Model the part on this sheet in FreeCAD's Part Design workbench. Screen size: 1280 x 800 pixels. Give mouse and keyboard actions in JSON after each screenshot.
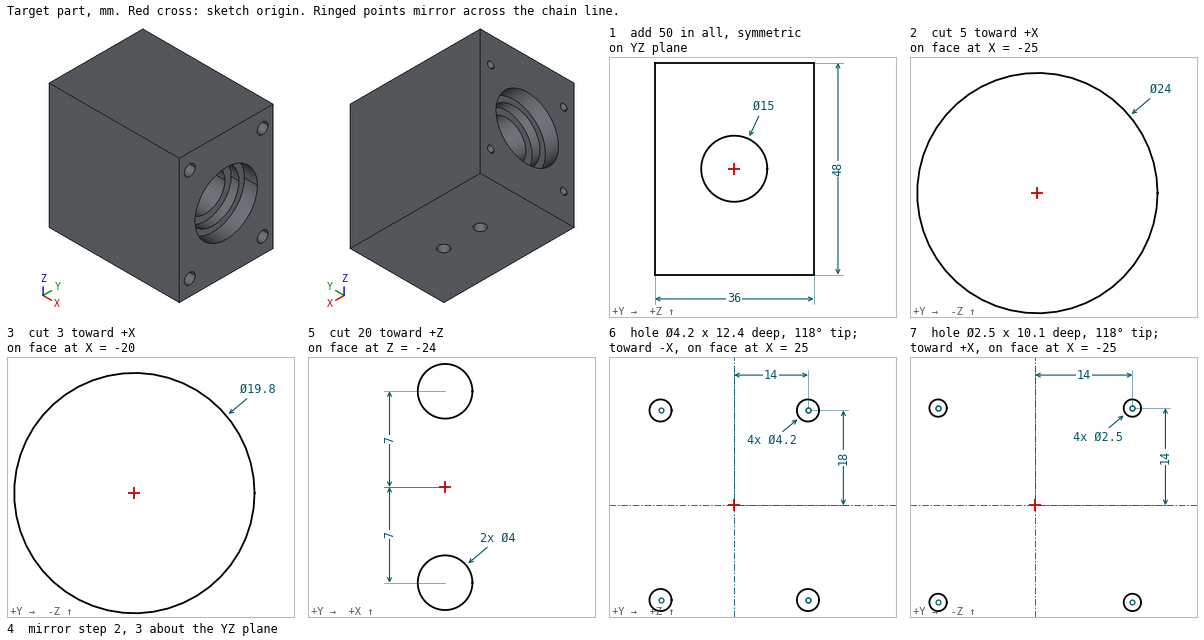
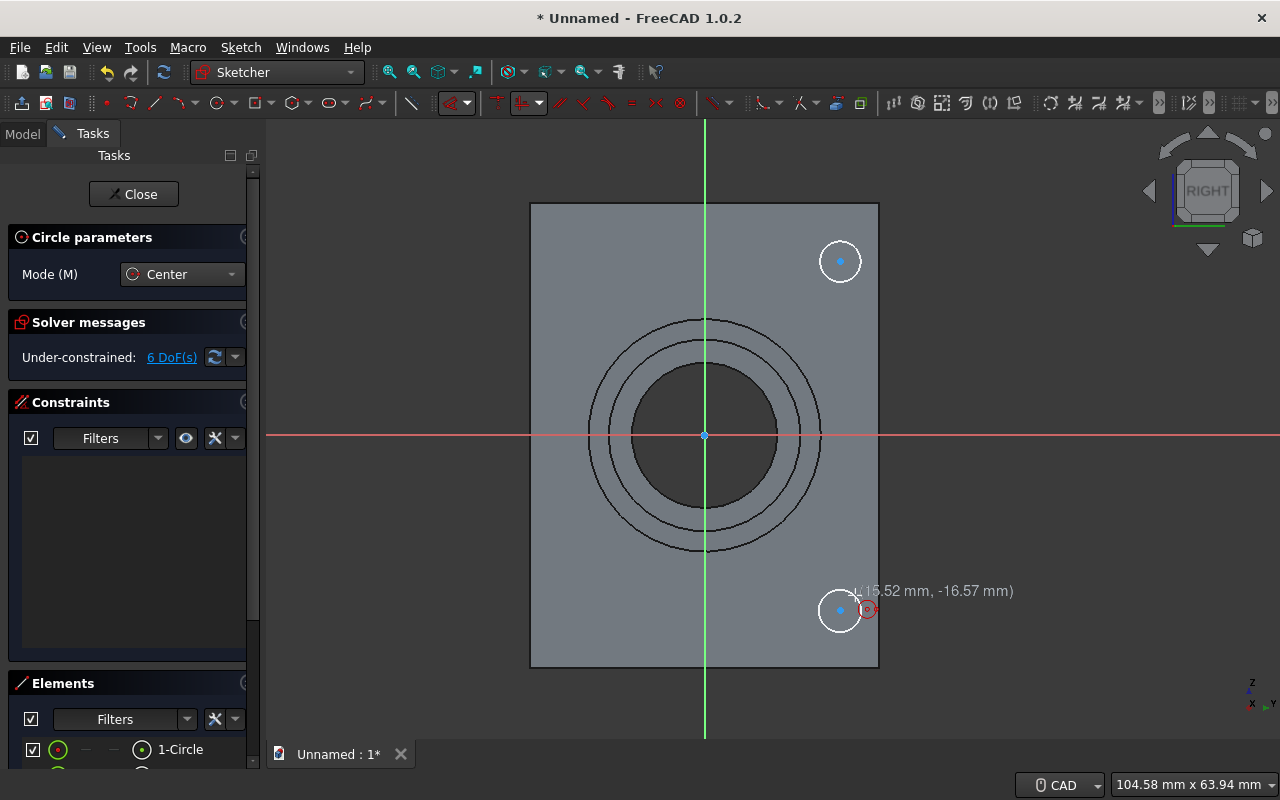
{"action": "left_click", "coordinate": [569, 261]}
{"action": "left_click", "coordinate": [583, 246]}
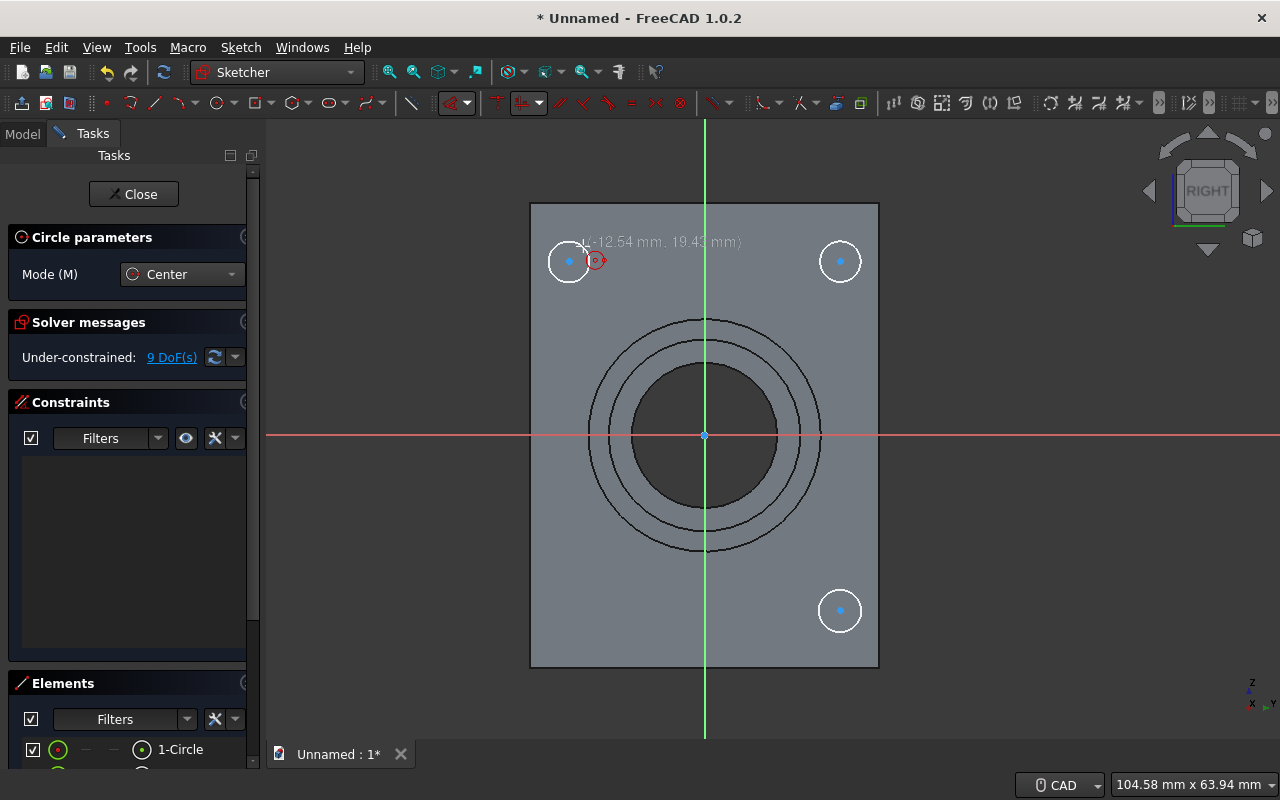
{"action": "left_click", "coordinate": [569, 610]}
{"action": "left_click", "coordinate": [583, 595]}
{"action": "key", "text": "Escape"}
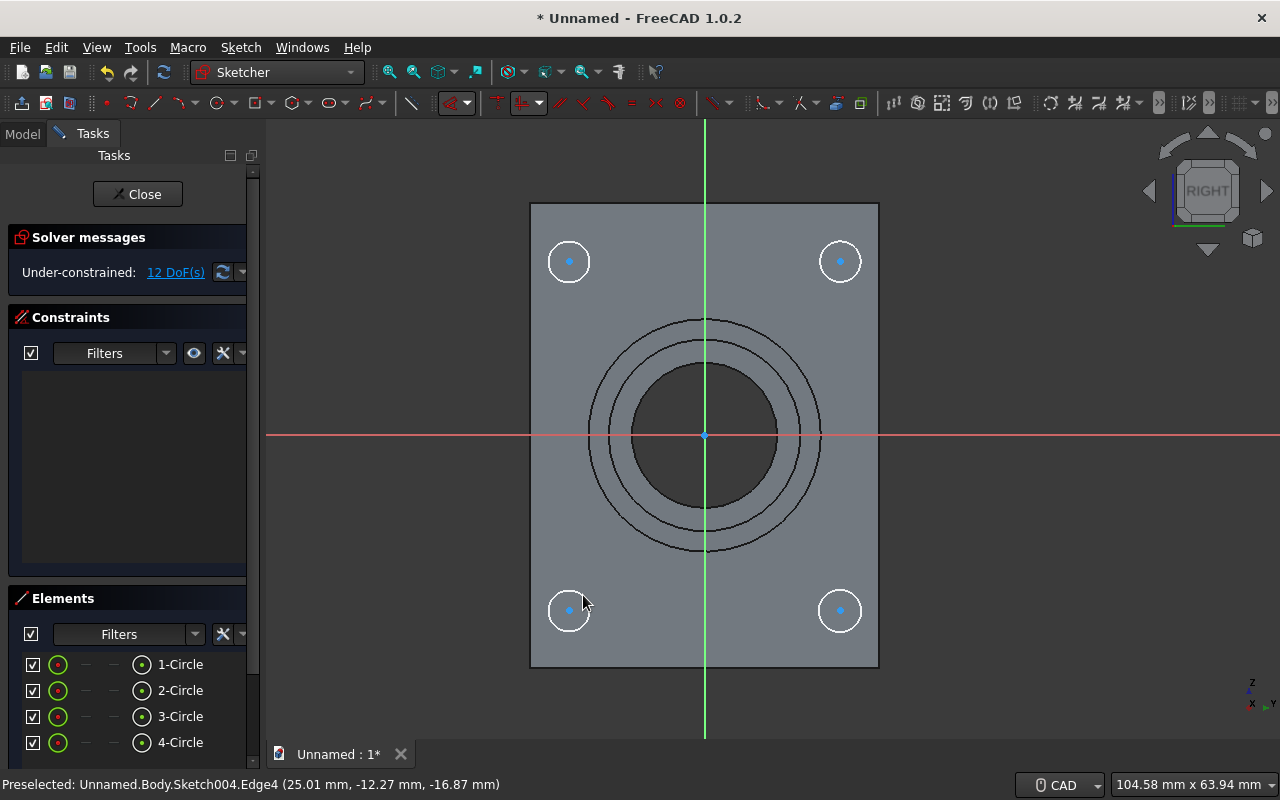
{"action": "left_click", "coordinate": [855, 247]}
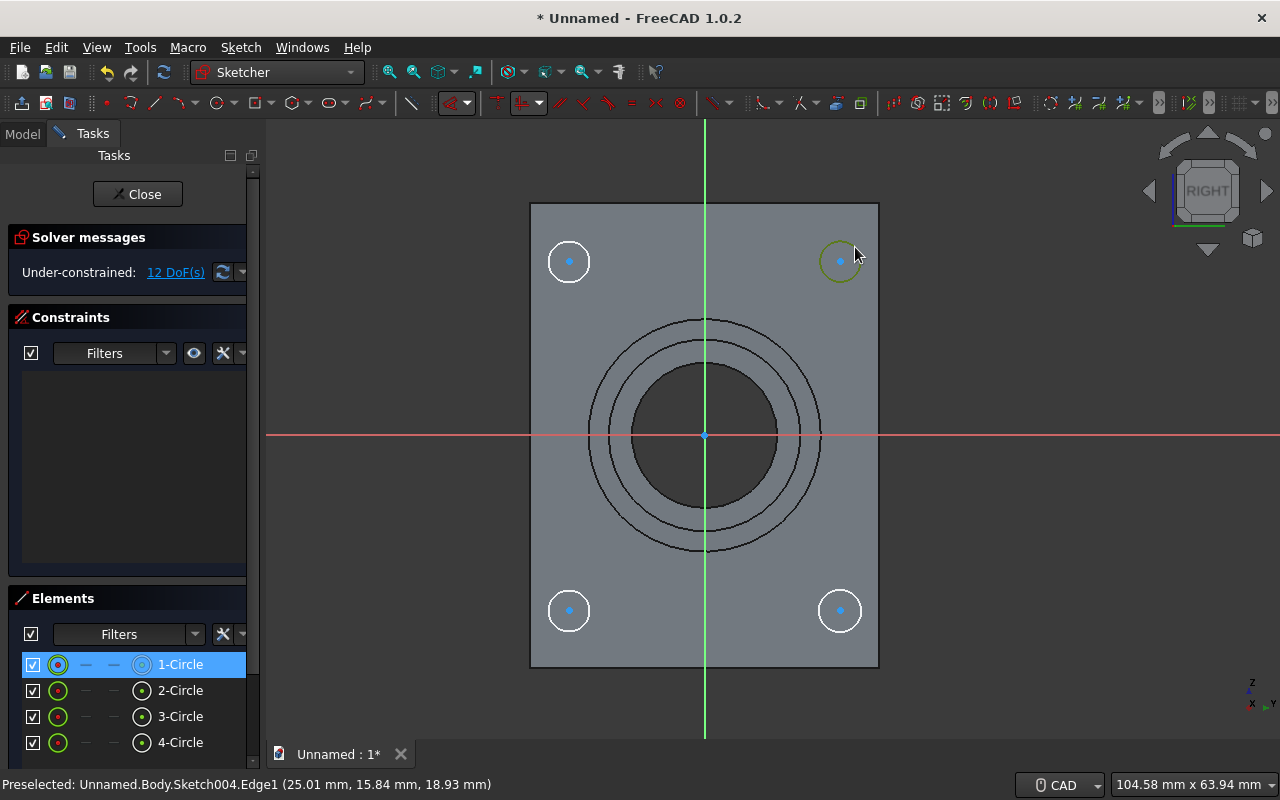
{"action": "left_click", "coordinate": [855, 596]}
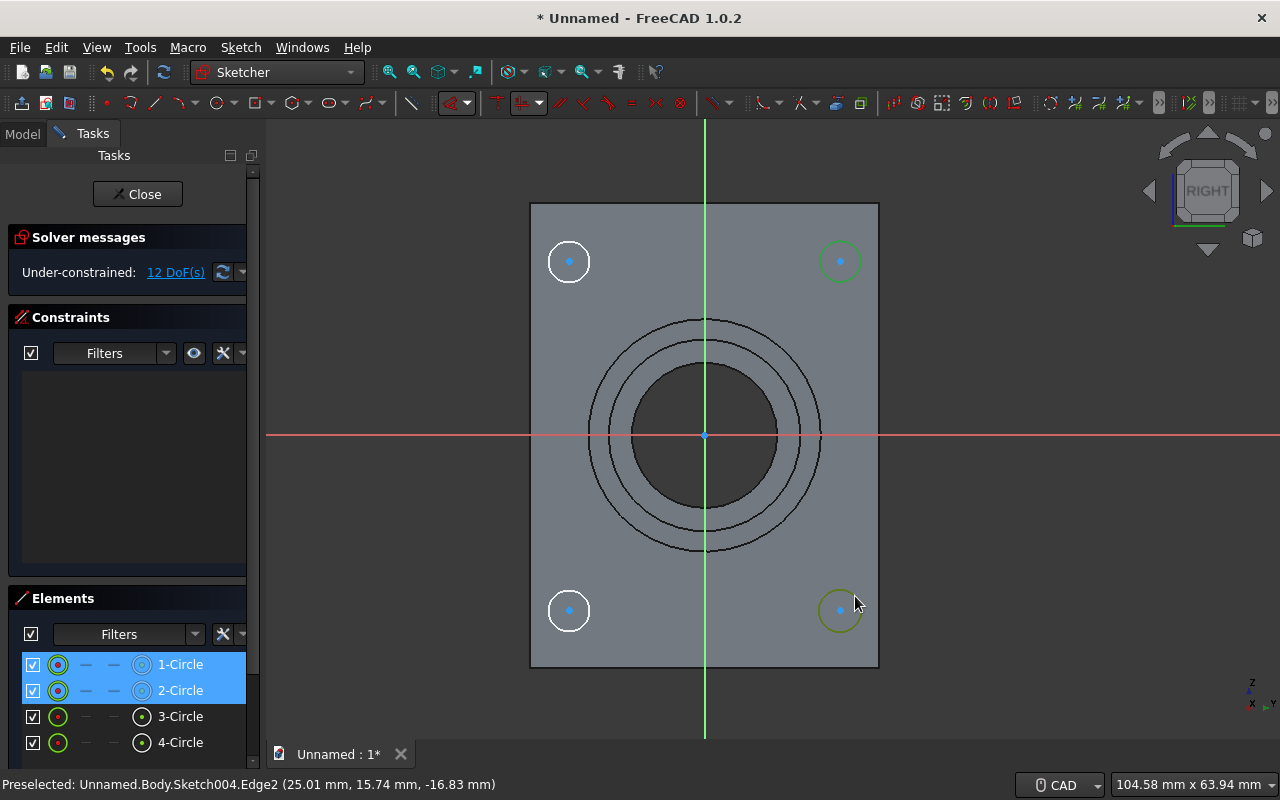
{"action": "left_click", "coordinate": [583, 247]}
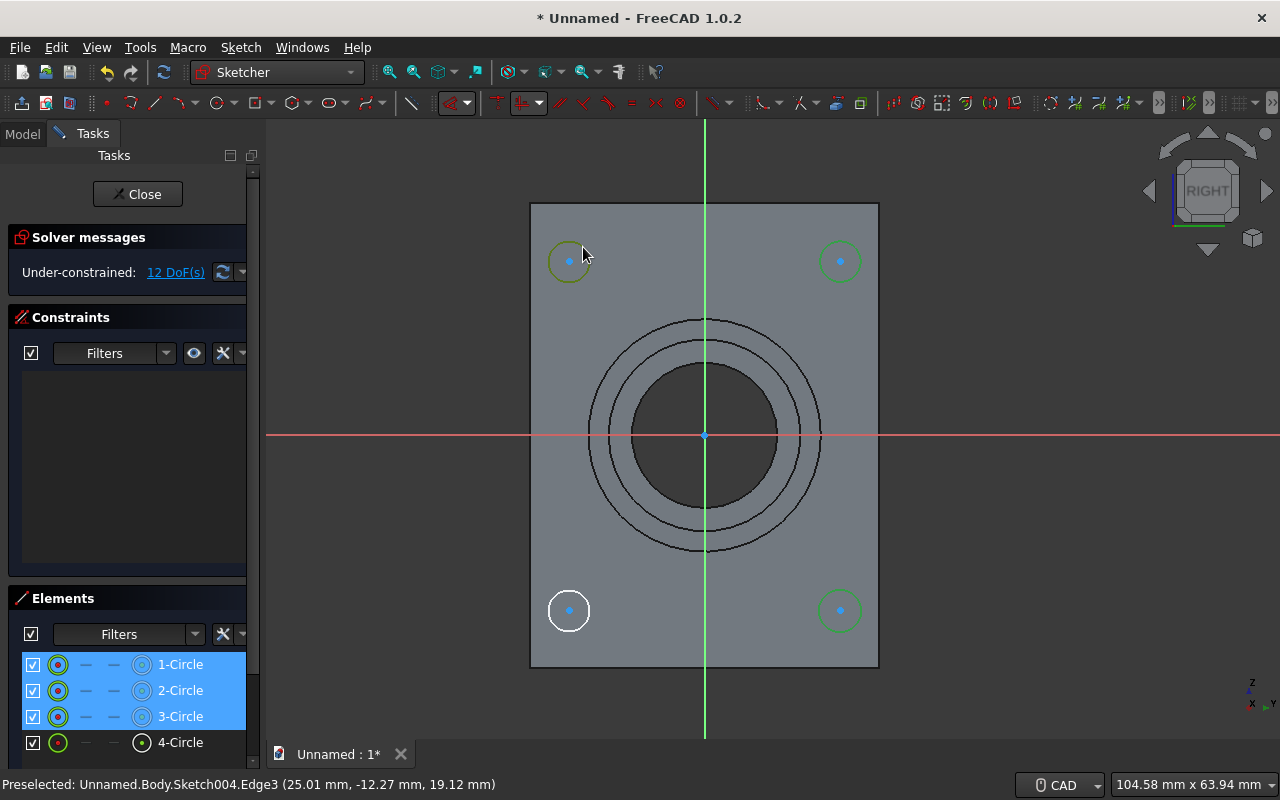
{"action": "left_click", "coordinate": [583, 596]}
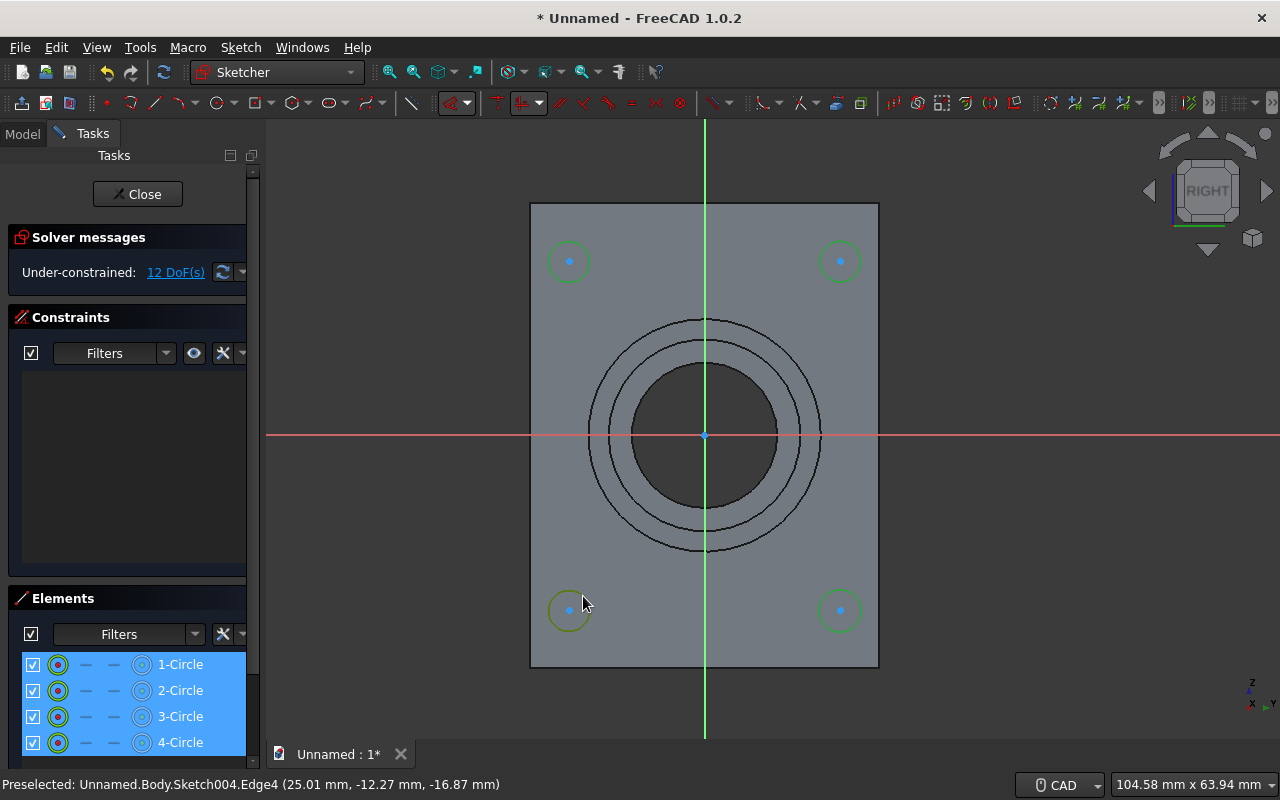
{"action": "left_click", "coordinate": [632, 104]}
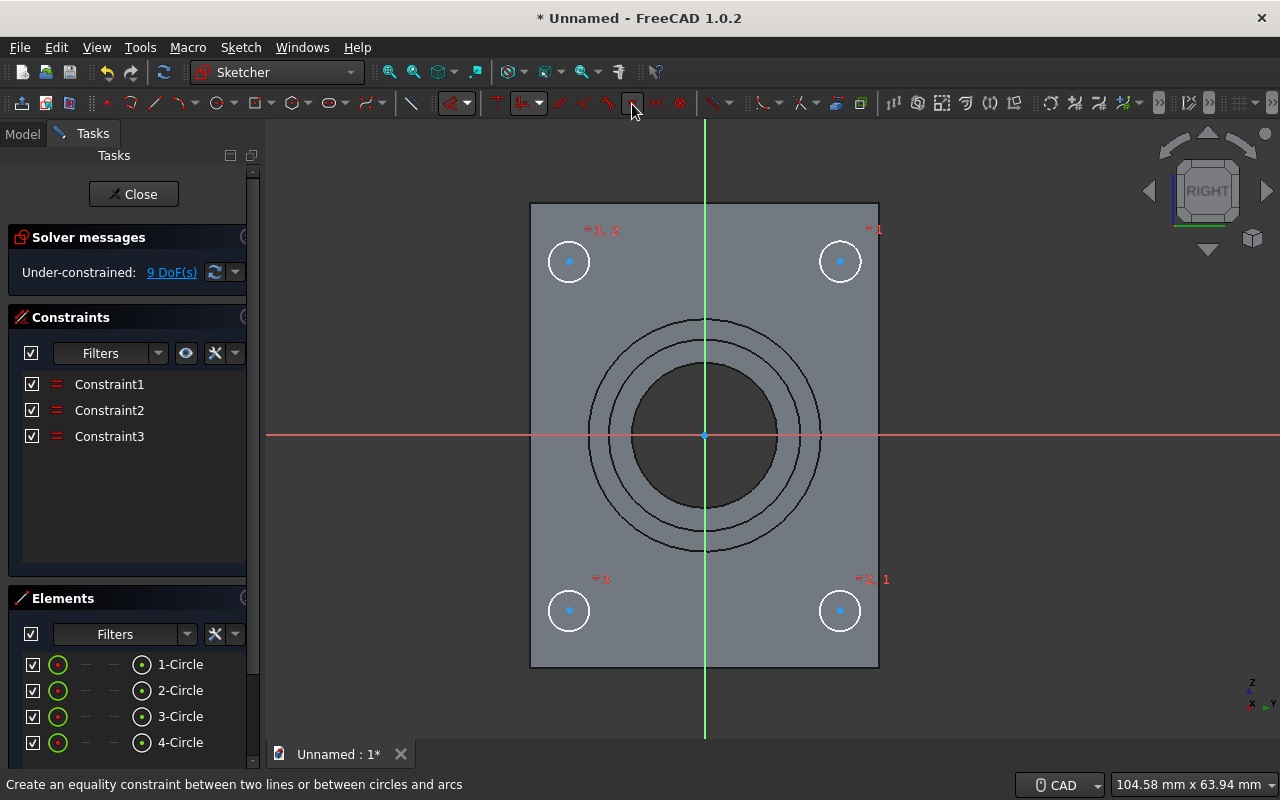
{"action": "left_click", "coordinate": [840, 262]}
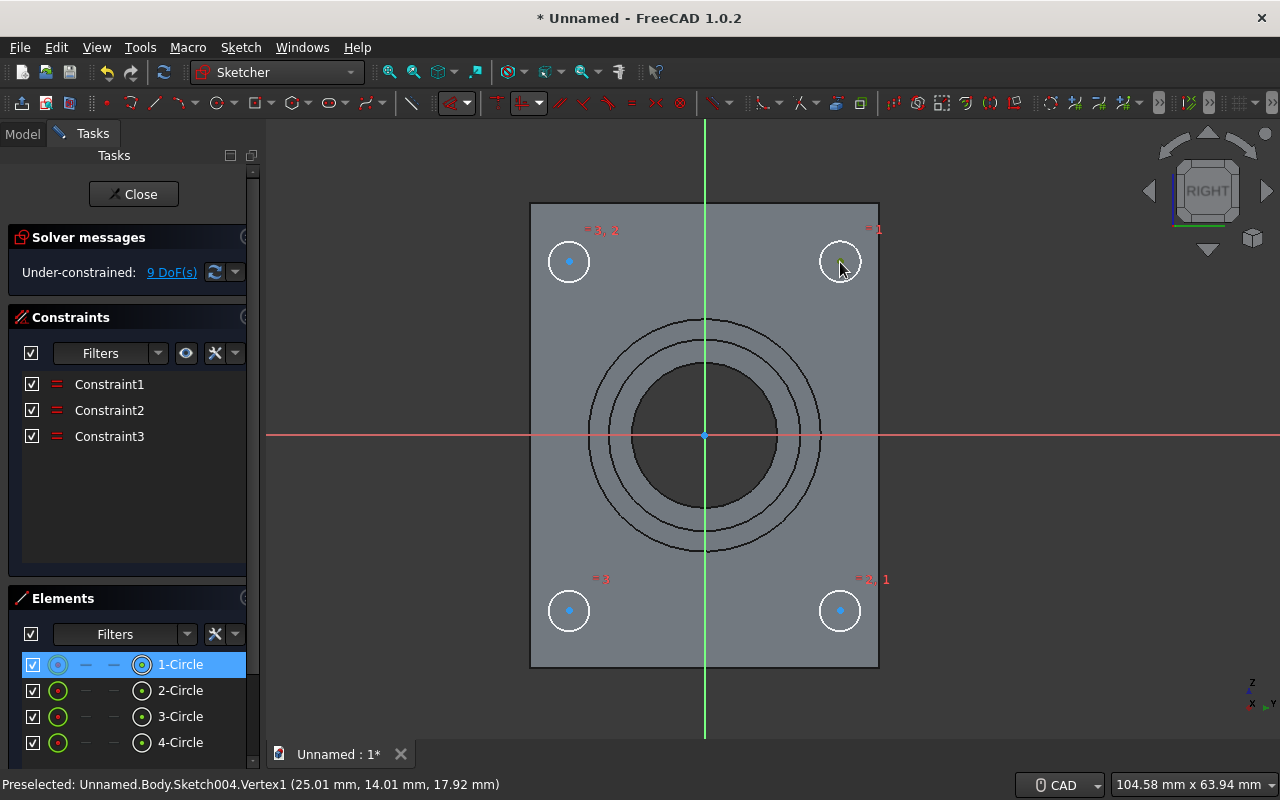
{"action": "left_click", "coordinate": [840, 611]}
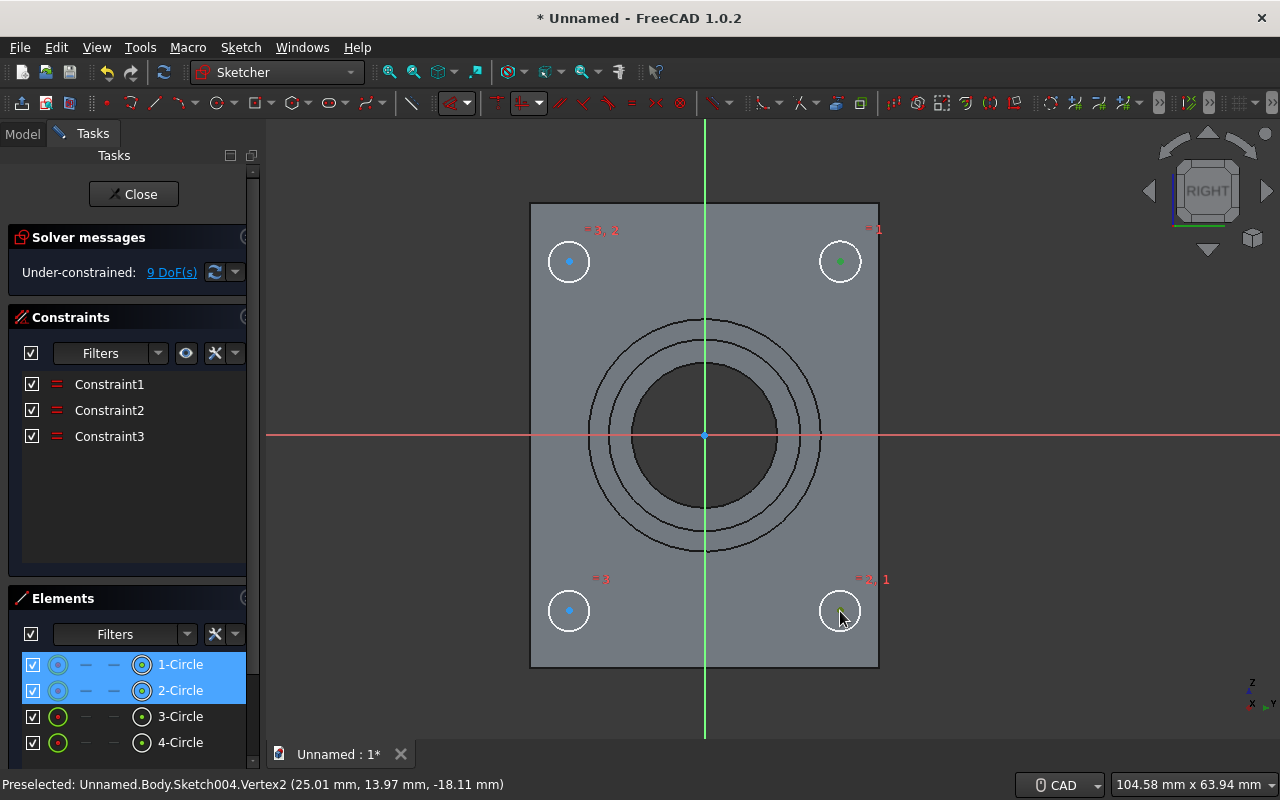
{"action": "left_click", "coordinate": [353, 435]}